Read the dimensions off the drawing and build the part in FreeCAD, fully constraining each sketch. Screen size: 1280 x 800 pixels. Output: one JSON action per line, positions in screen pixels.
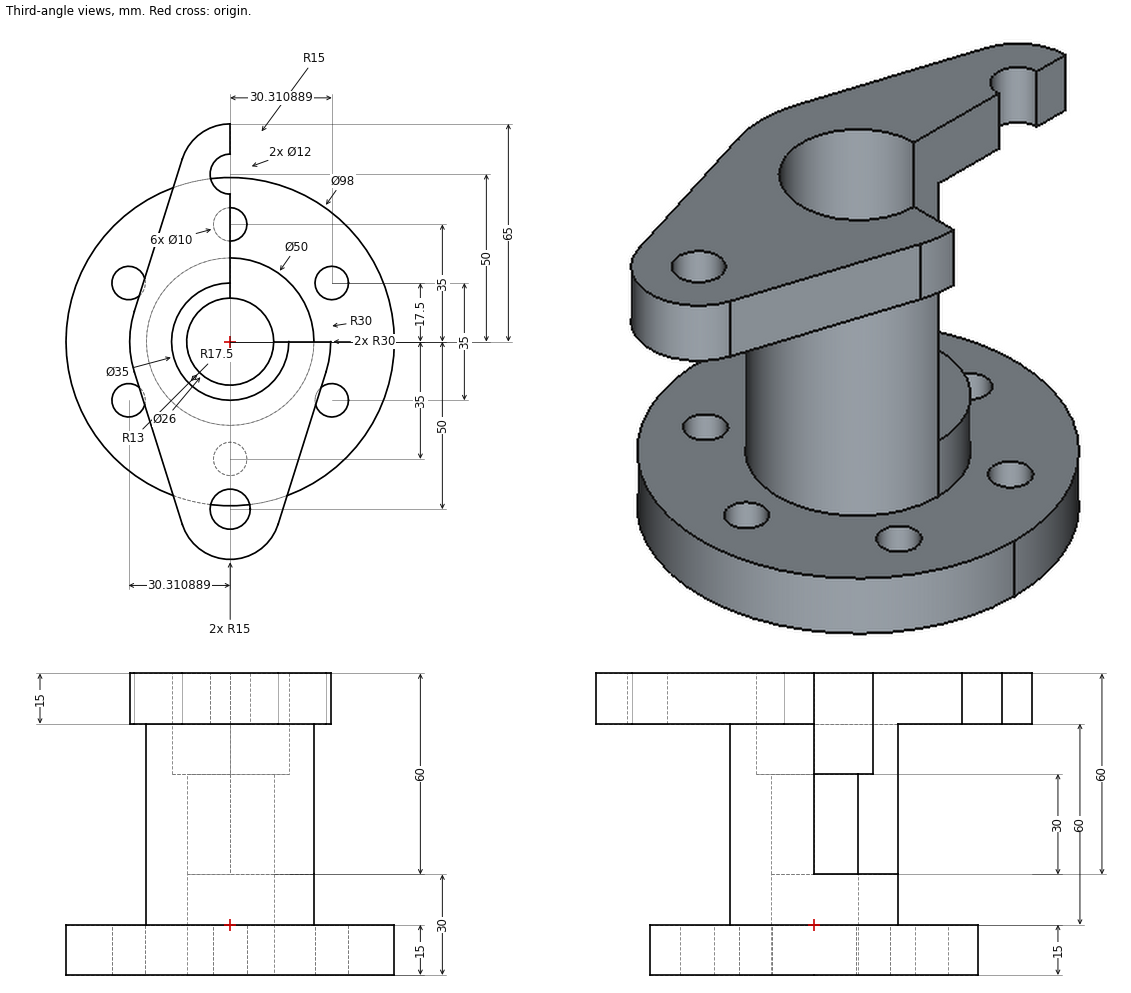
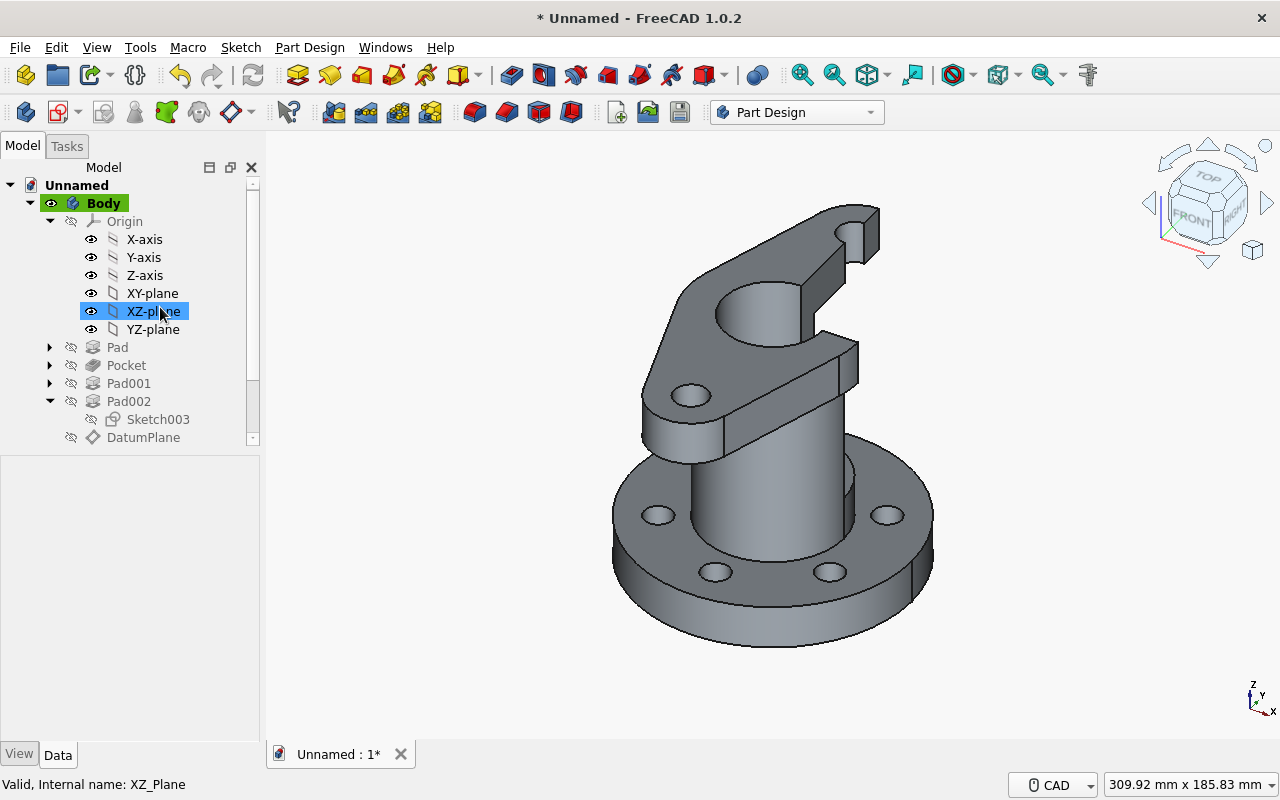
{"action": "left_click", "coordinate": [136, 293]}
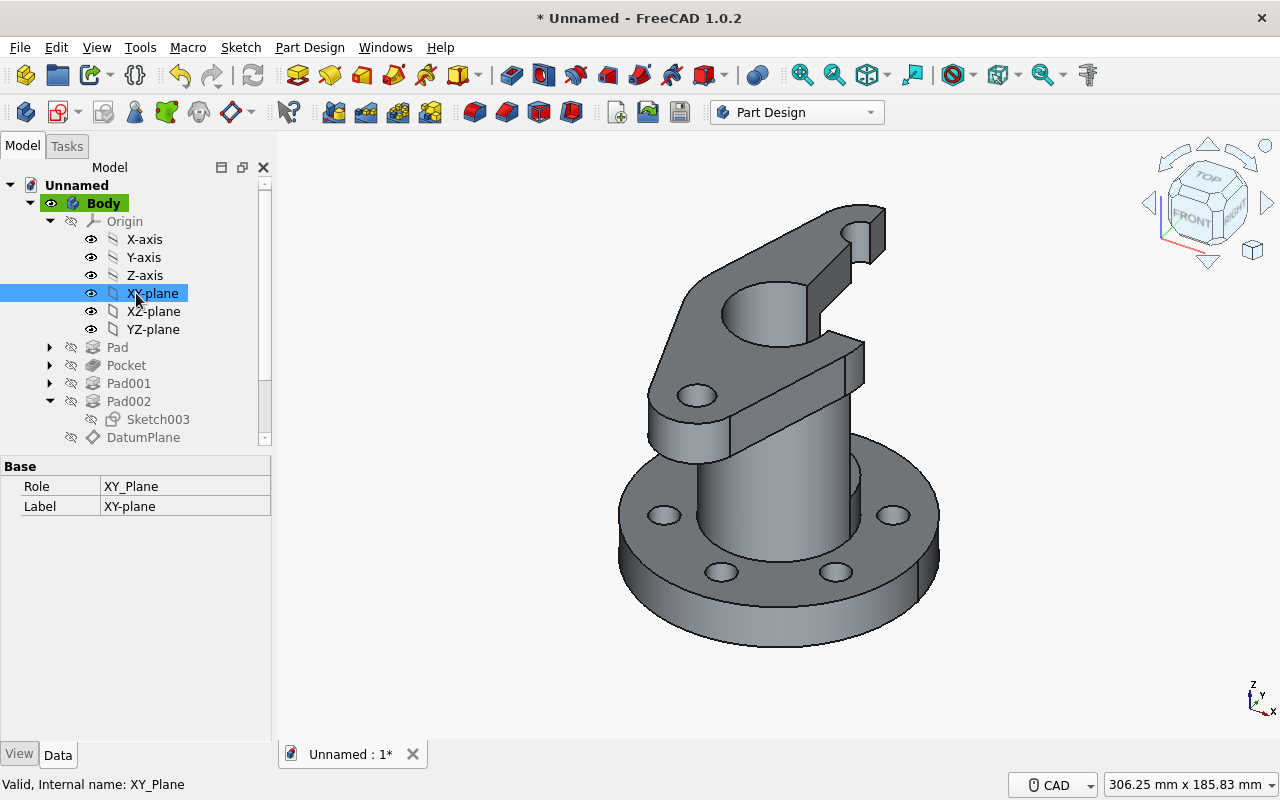
{"action": "left_click", "coordinate": [232, 112]}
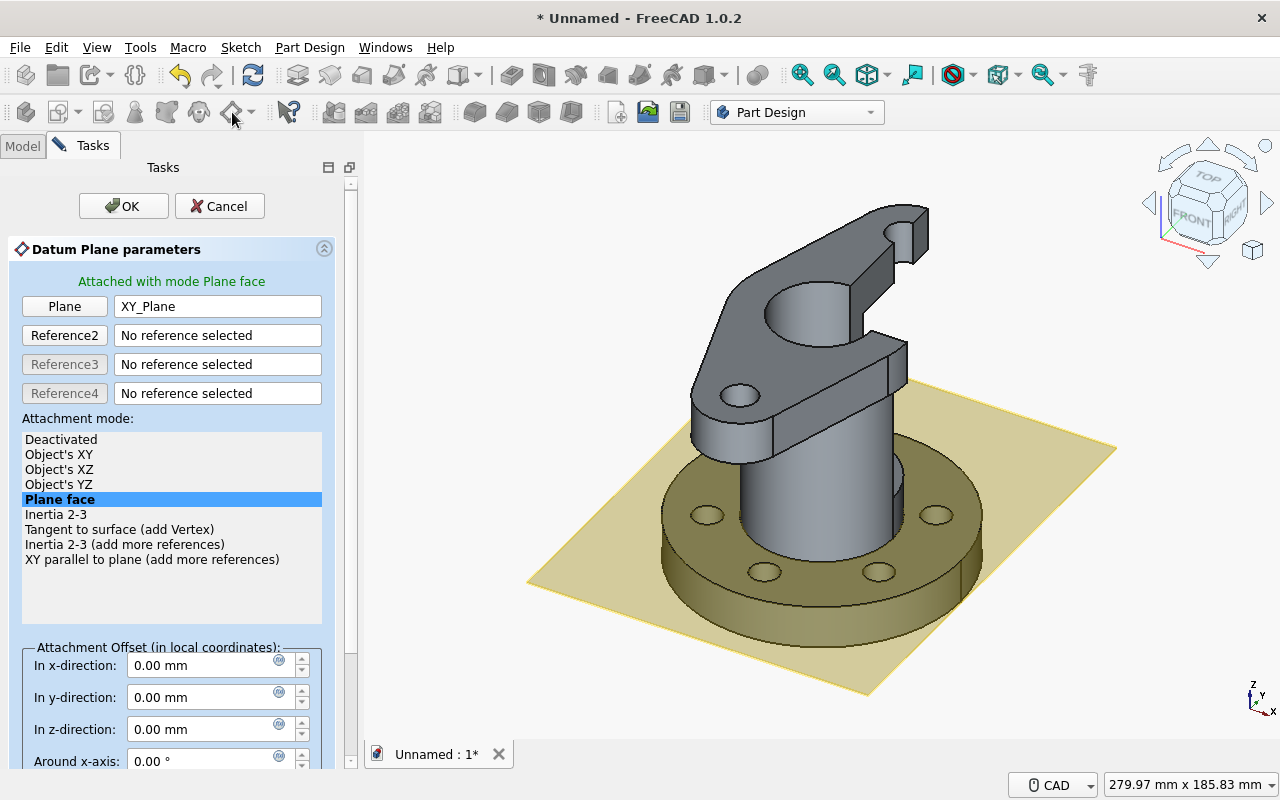
{"action": "triple_click", "coordinate": [210, 729]}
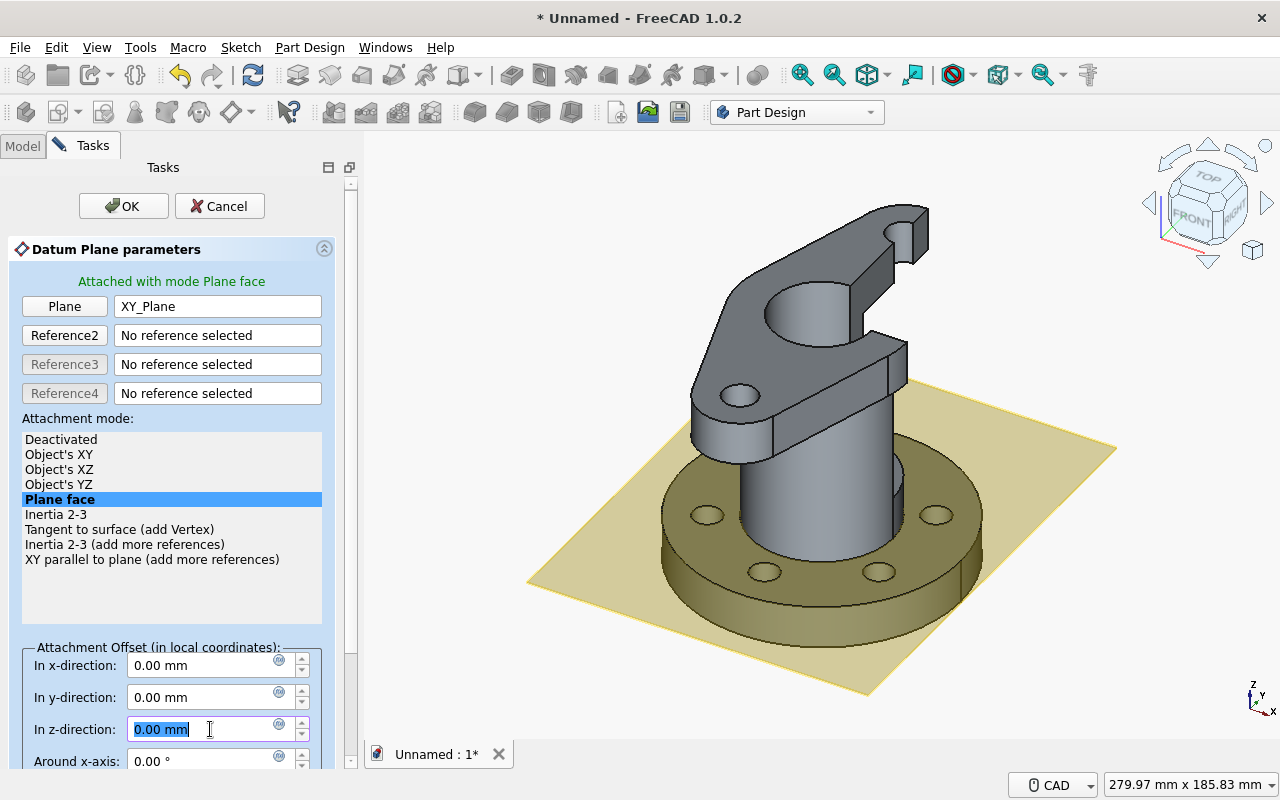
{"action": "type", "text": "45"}
{"action": "key", "text": "Tab"}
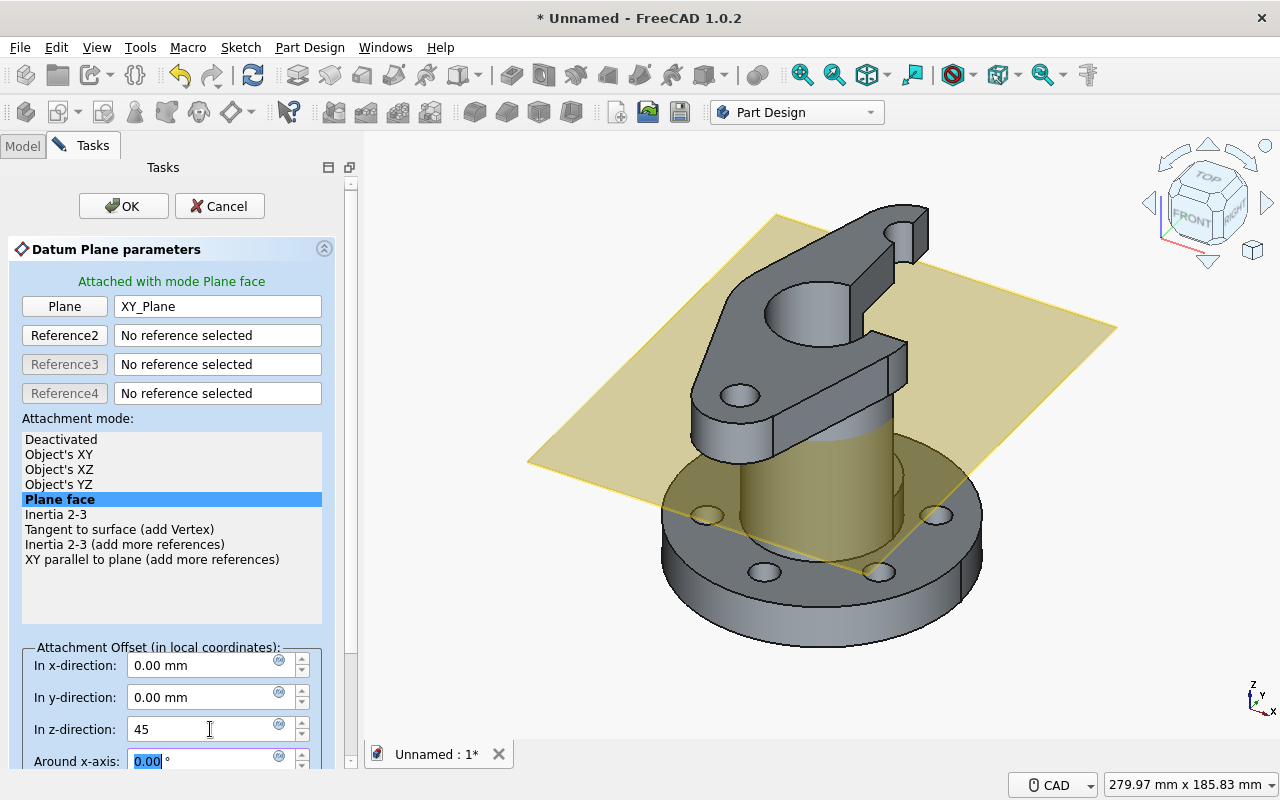
{"action": "left_click", "coordinate": [124, 206]}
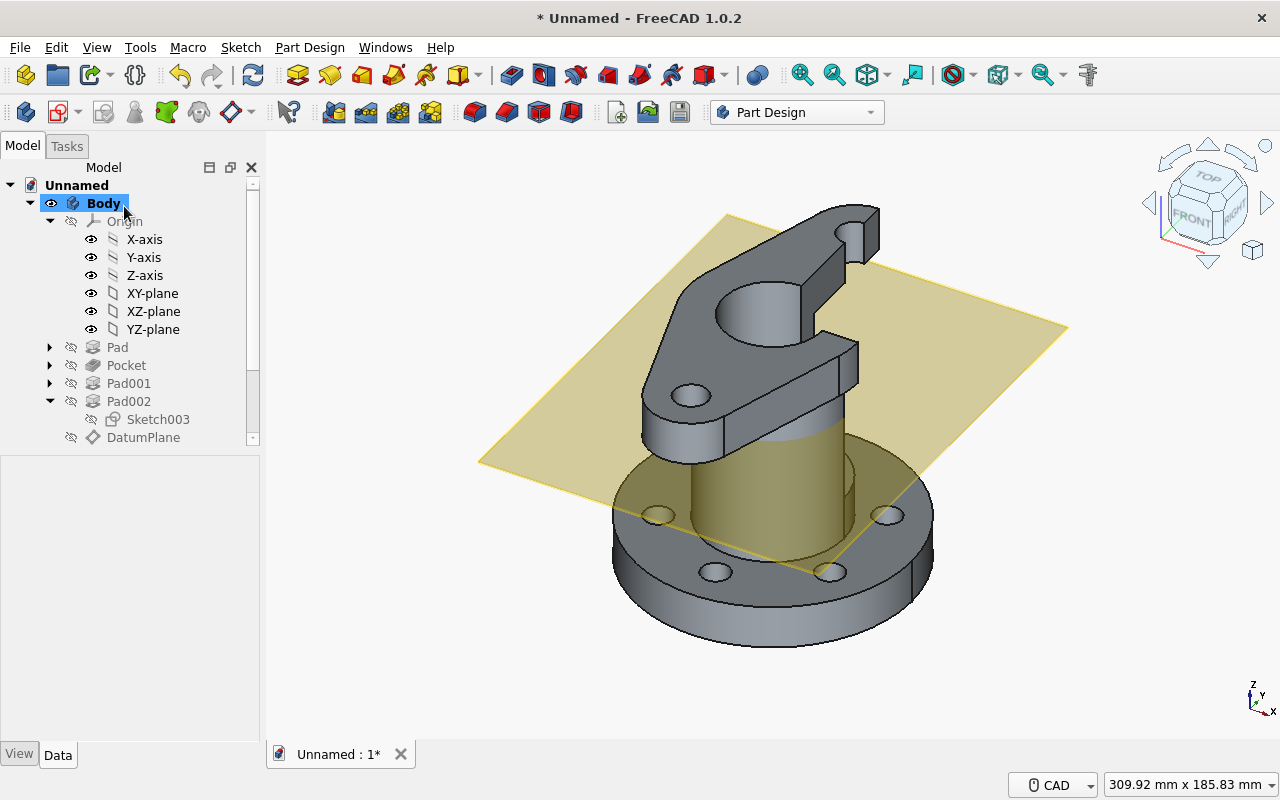
{"action": "scroll", "coordinate": [100, 307], "scroll_direction": "down", "scroll_amount": 3}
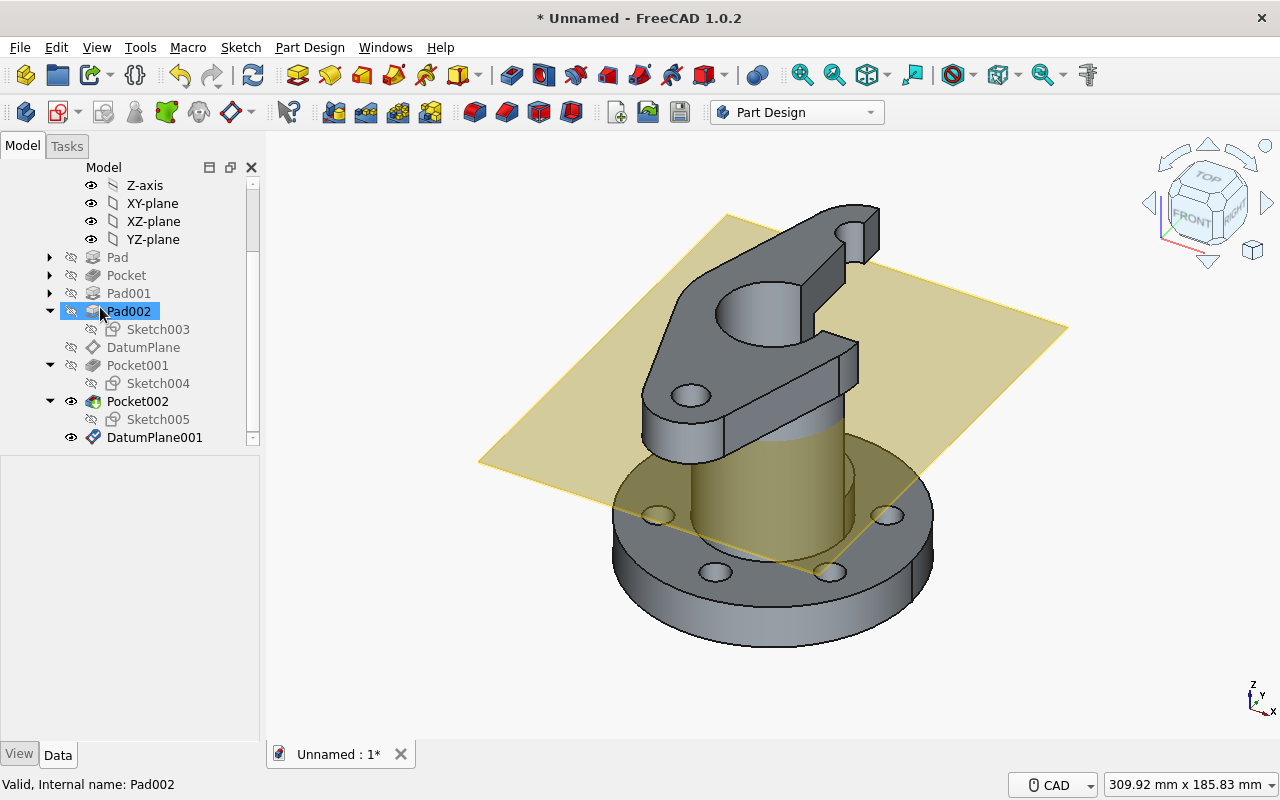
{"action": "left_click", "coordinate": [116, 437]}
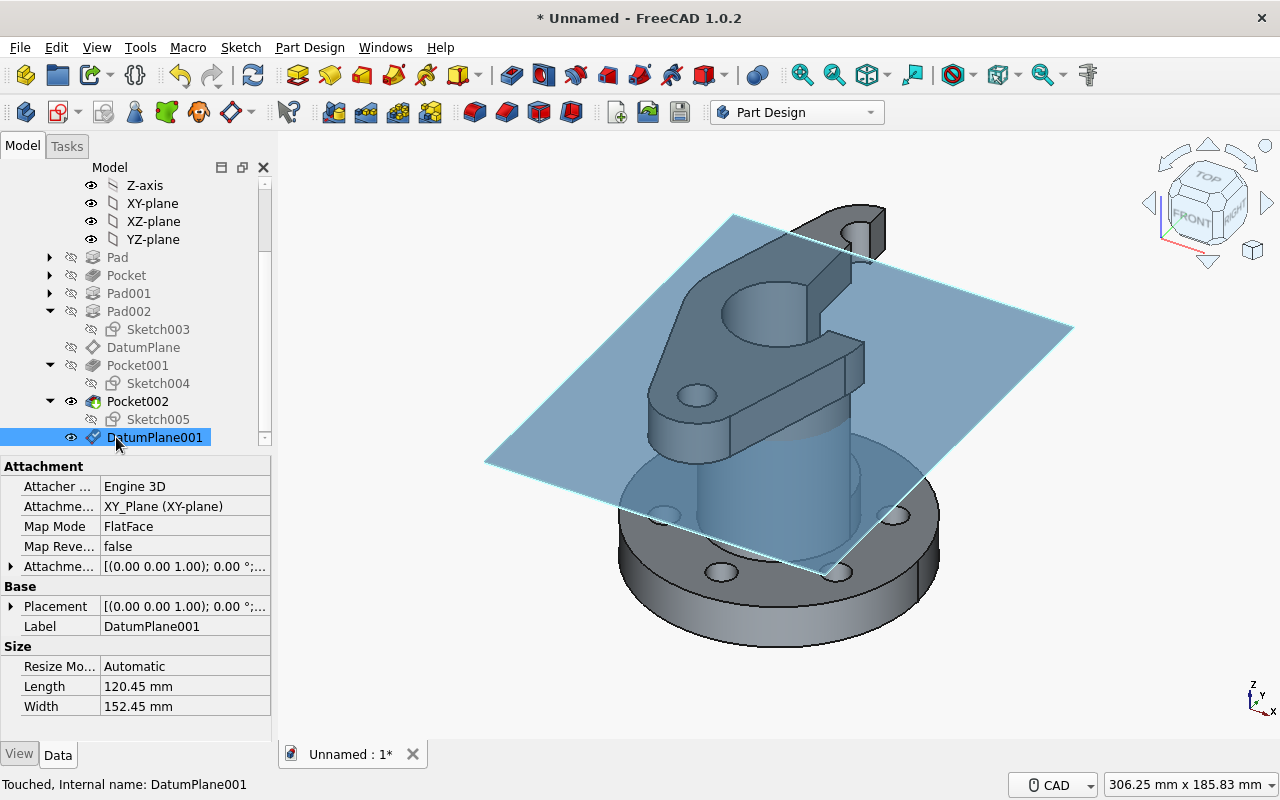
{"action": "left_click", "coordinate": [58, 112]}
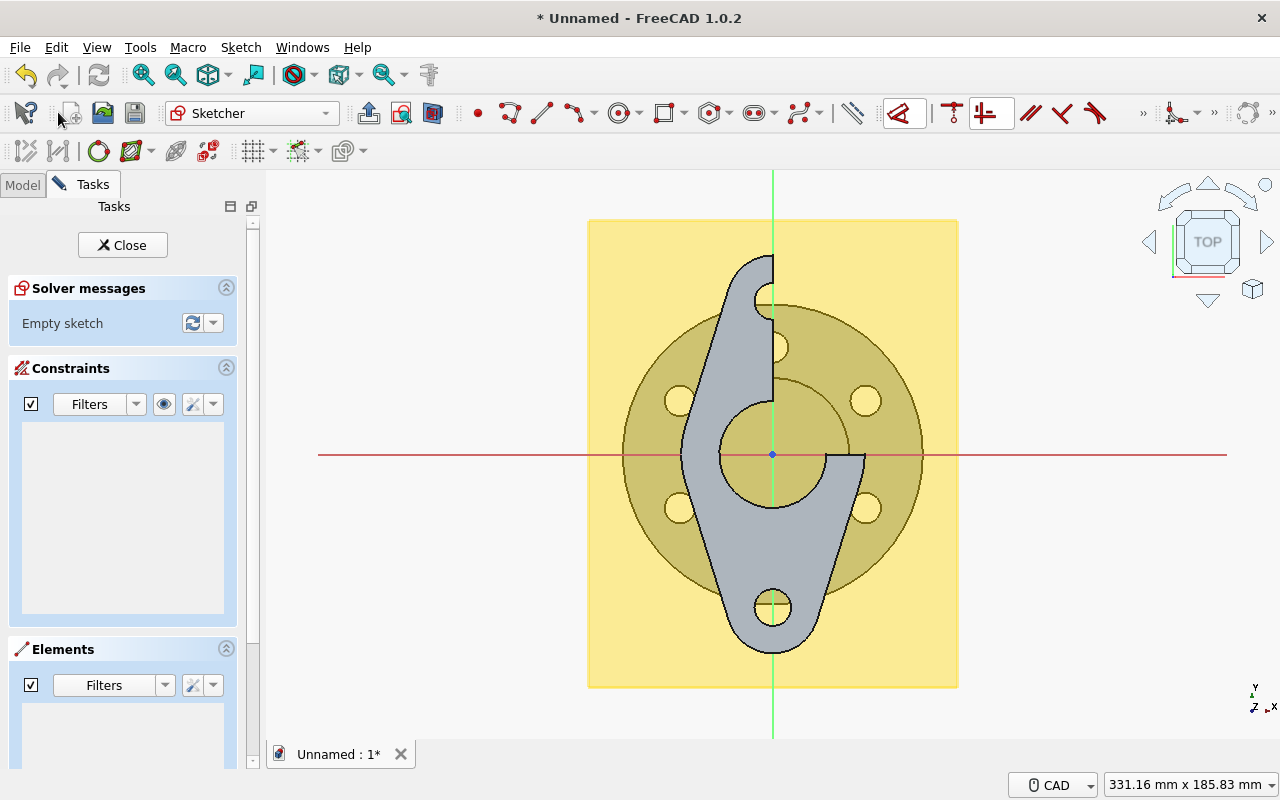
{"action": "left_click", "coordinate": [434, 114]}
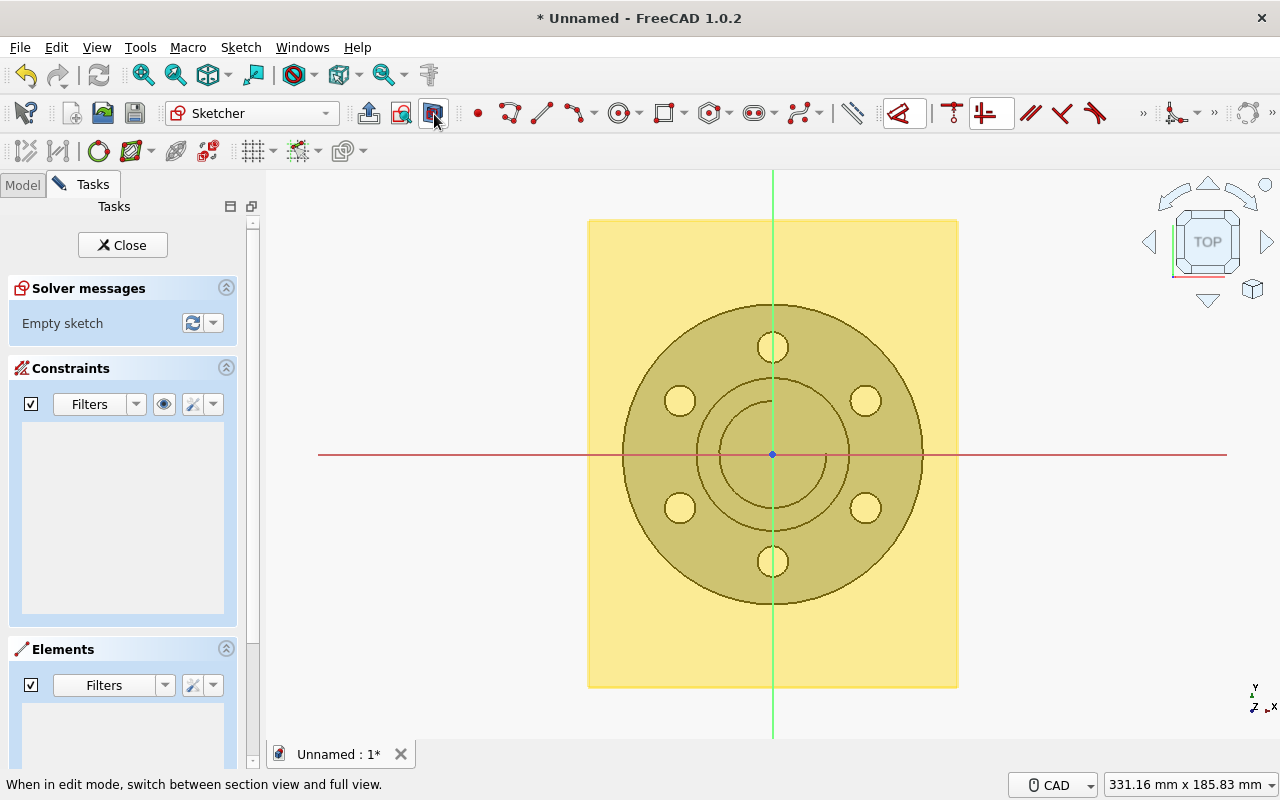
{"action": "scroll", "coordinate": [806, 444], "scroll_direction": "up", "scroll_amount": 7}